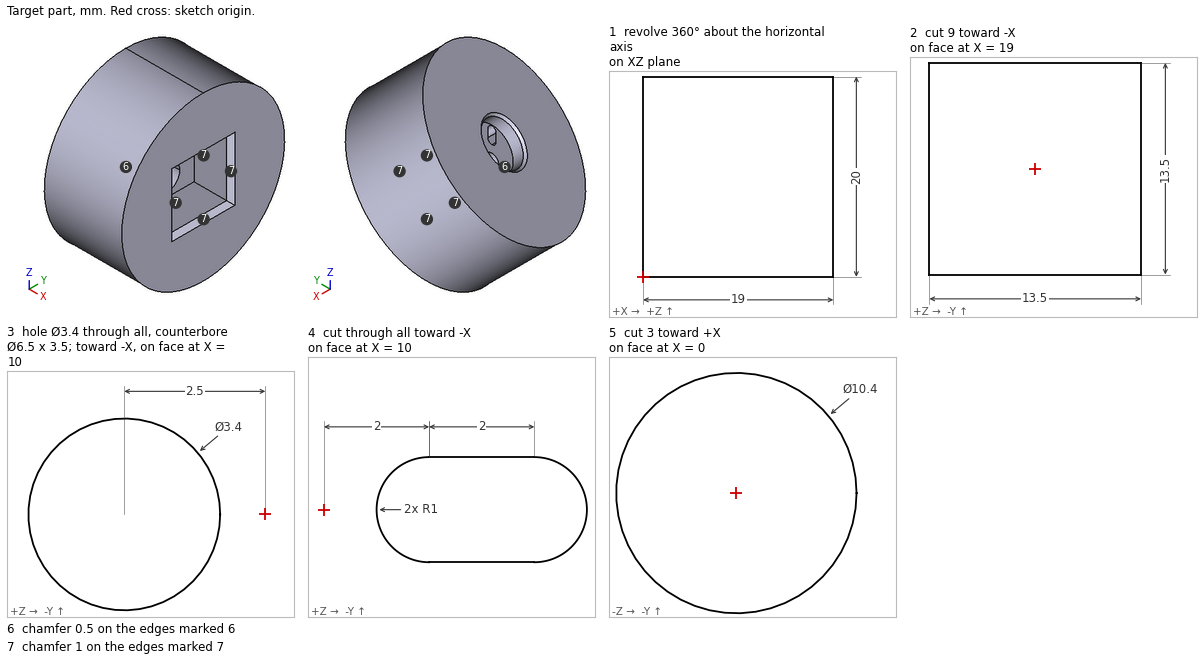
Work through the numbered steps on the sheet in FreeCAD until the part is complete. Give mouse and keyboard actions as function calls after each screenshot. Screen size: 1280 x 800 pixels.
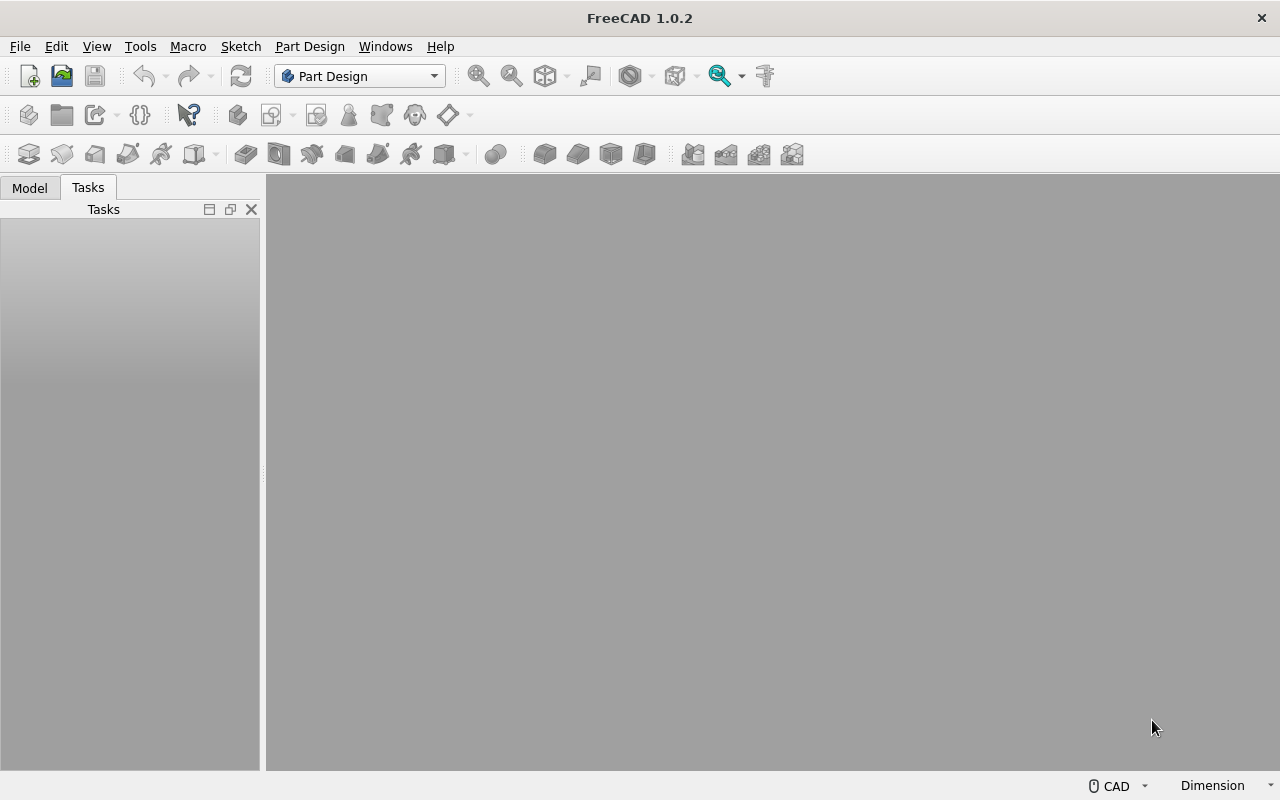
click(29, 76)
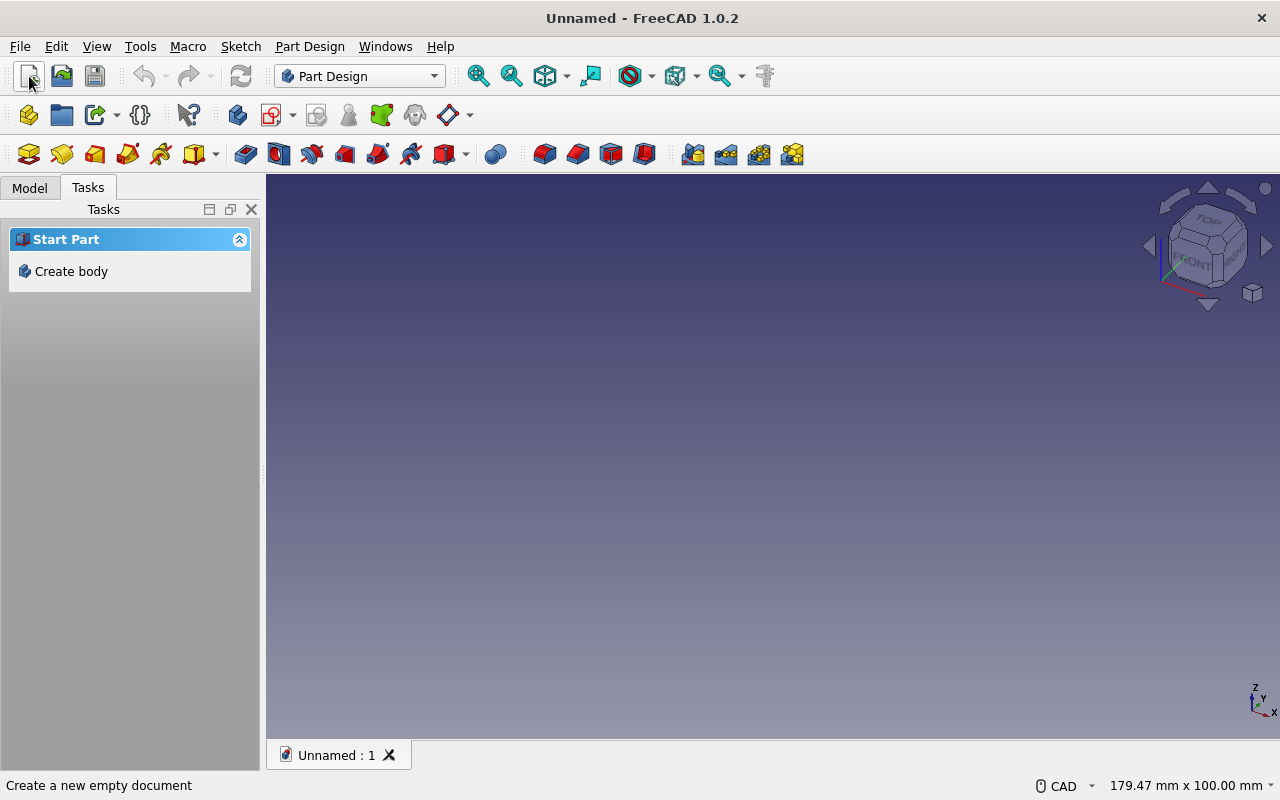
click(270, 116)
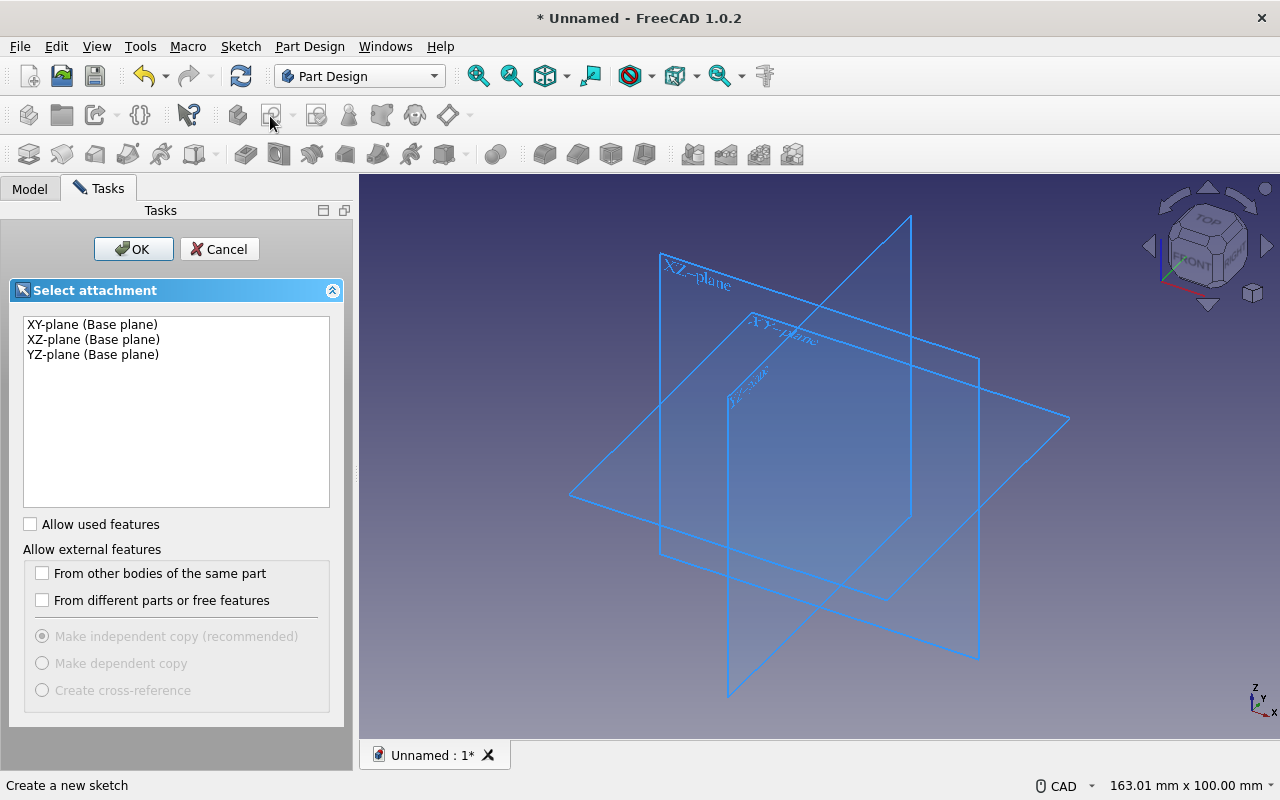
click(84, 340)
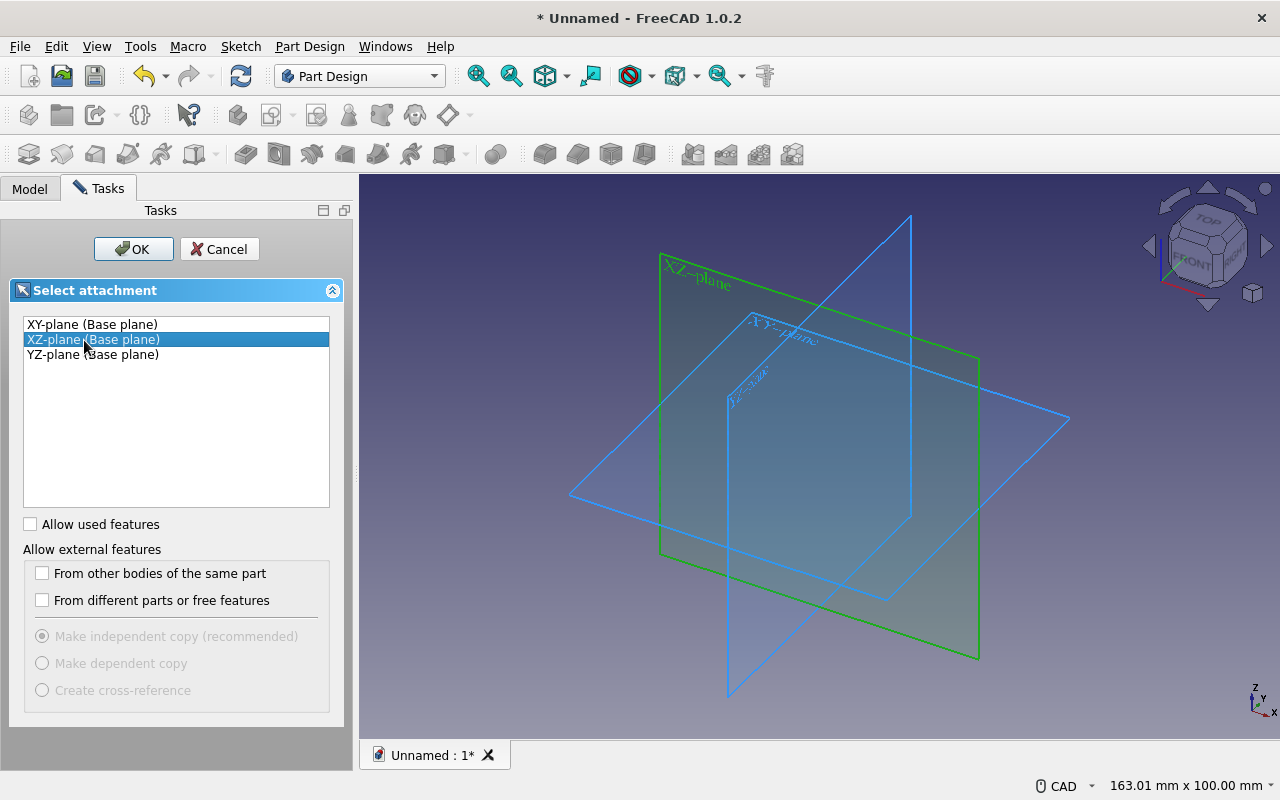
click(134, 249)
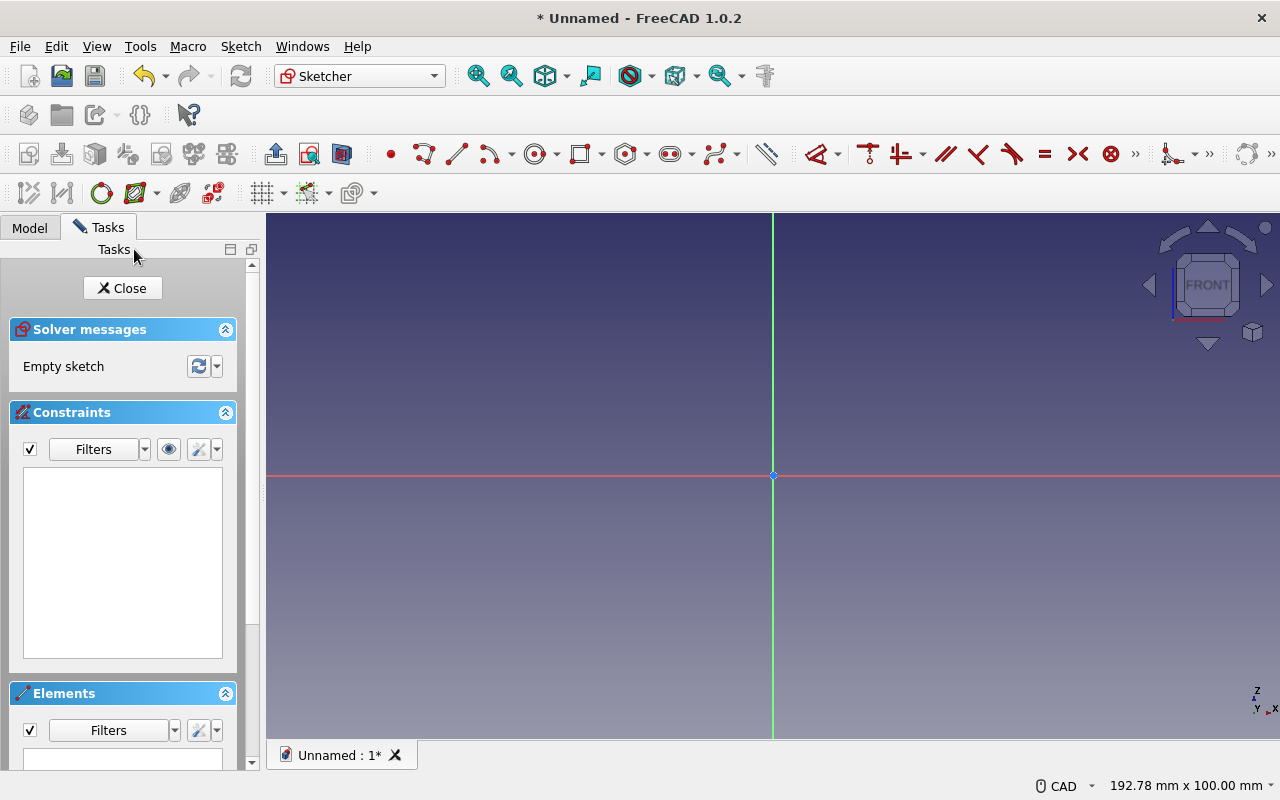
scroll(874, 401, up, 6)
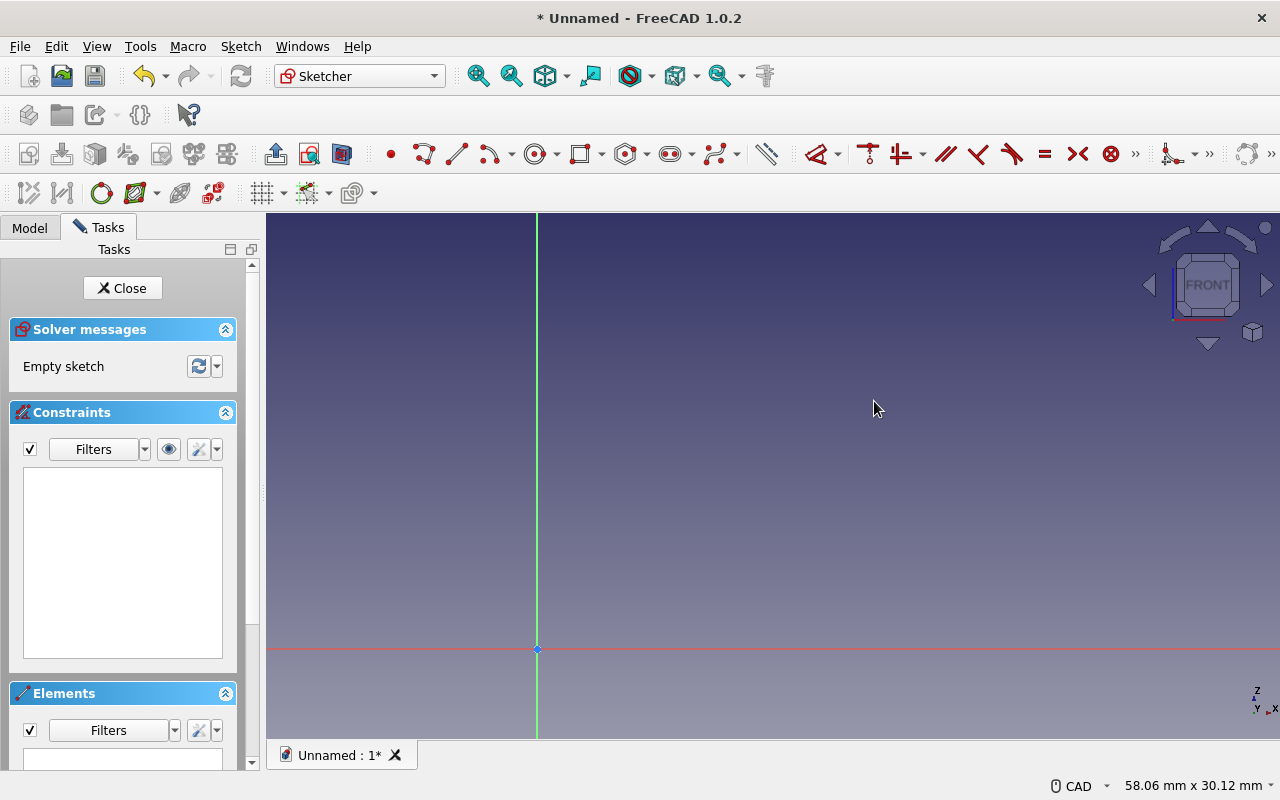
click(580, 154)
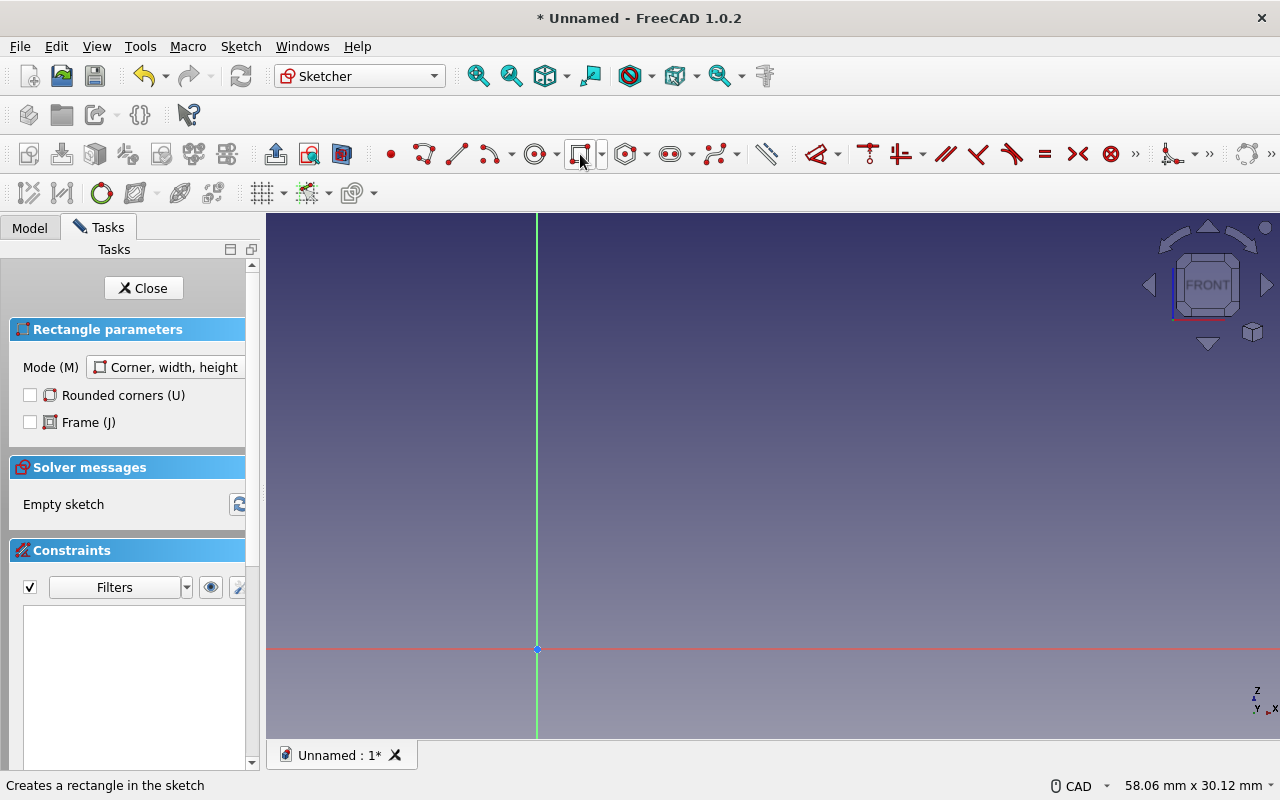
click(537, 649)
click(869, 300)
key(Escape)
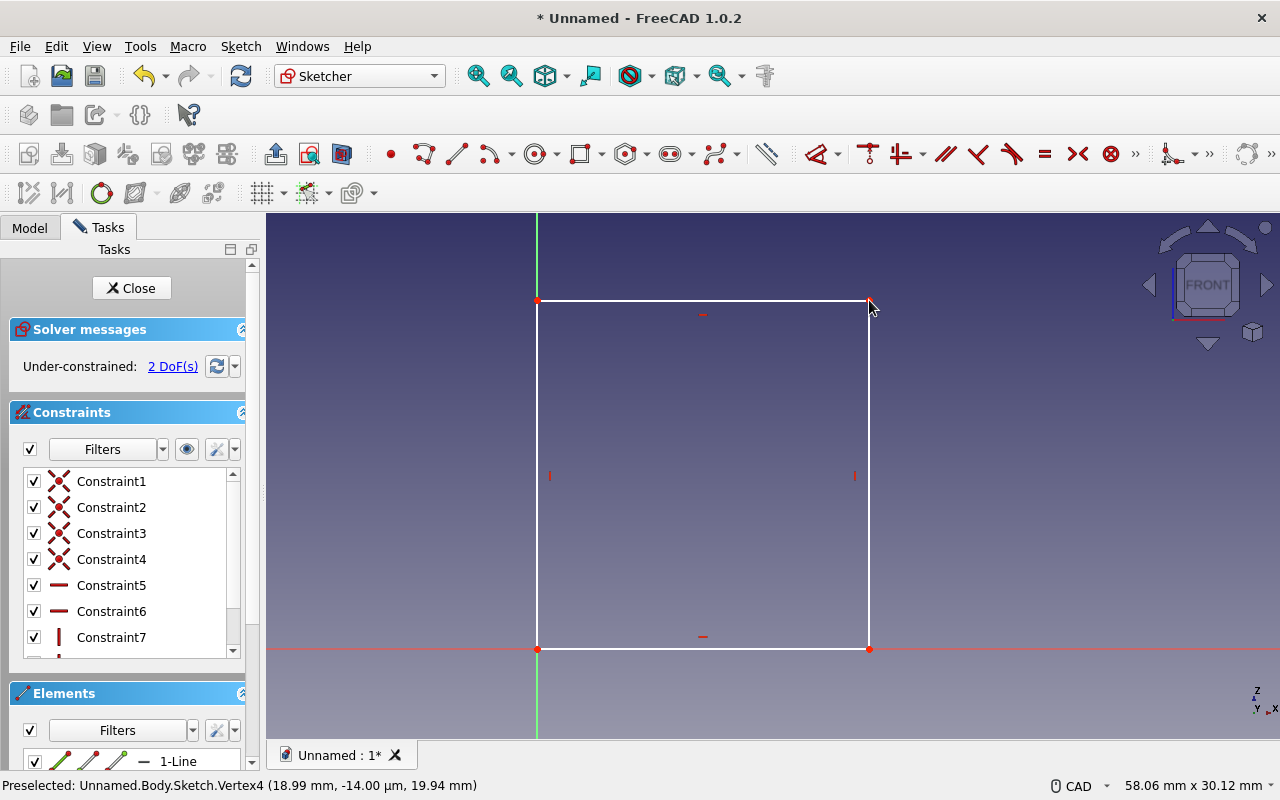
click(816, 154)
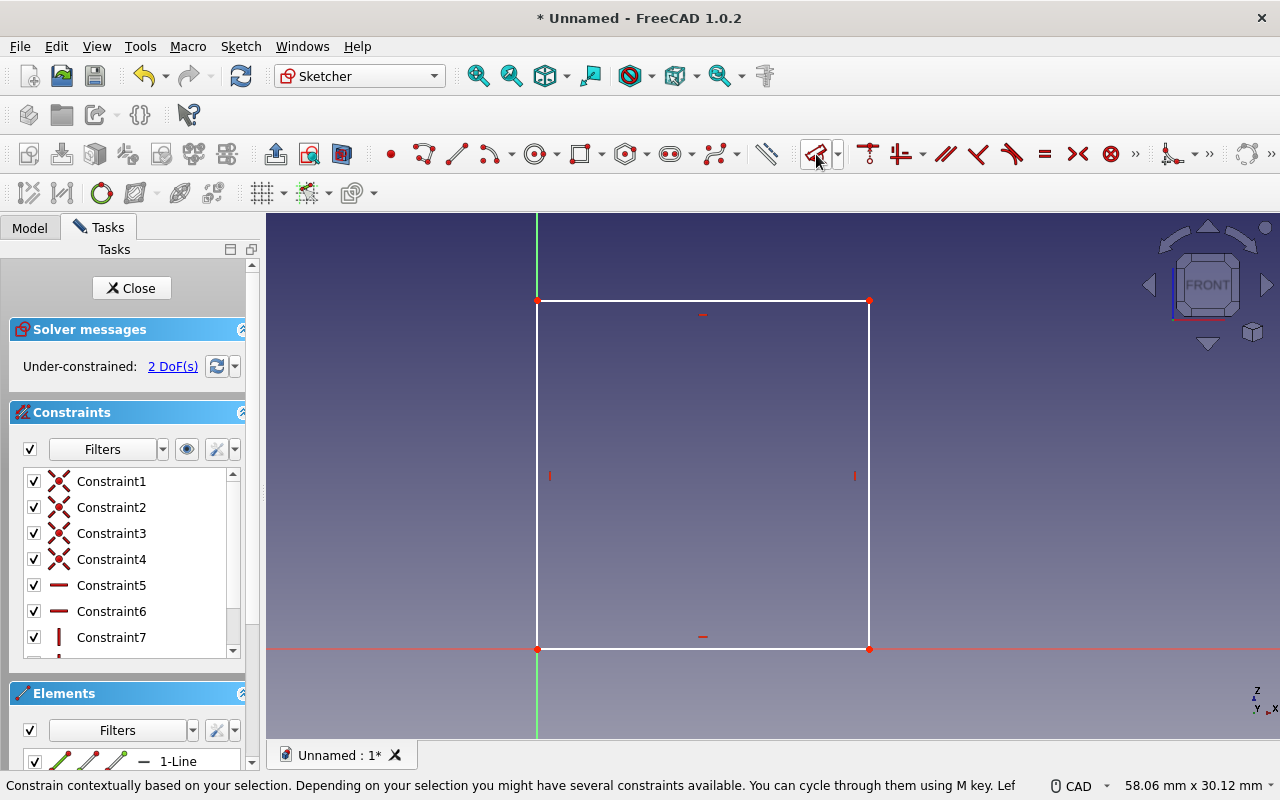
click(637, 649)
click(703, 683)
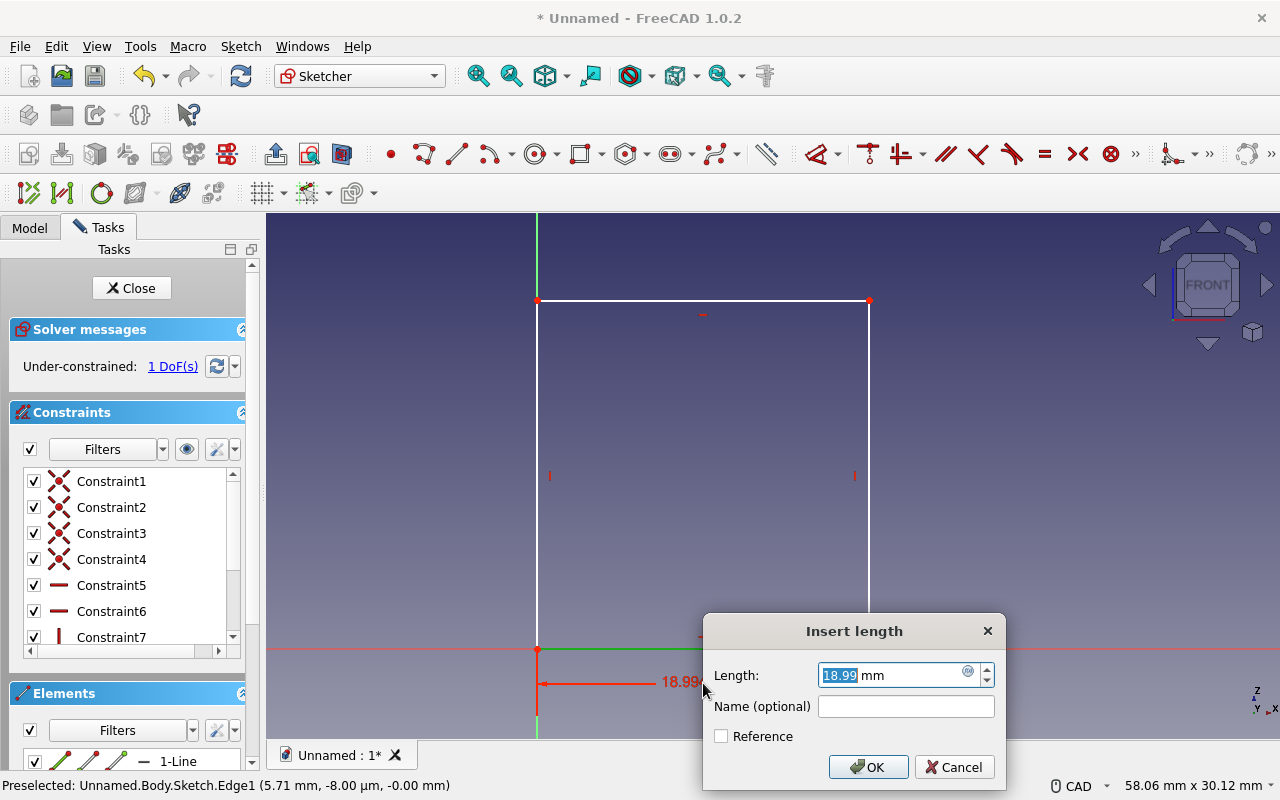
text(19)
key(Return)